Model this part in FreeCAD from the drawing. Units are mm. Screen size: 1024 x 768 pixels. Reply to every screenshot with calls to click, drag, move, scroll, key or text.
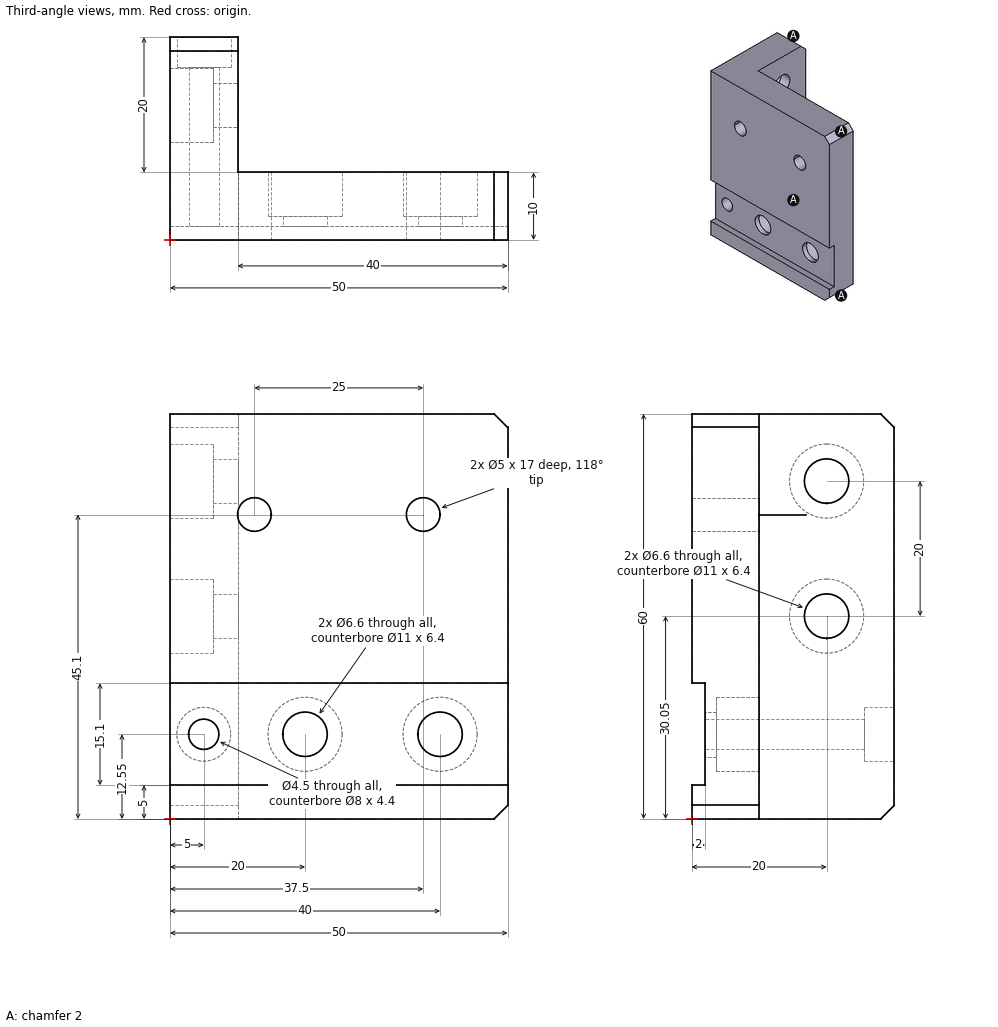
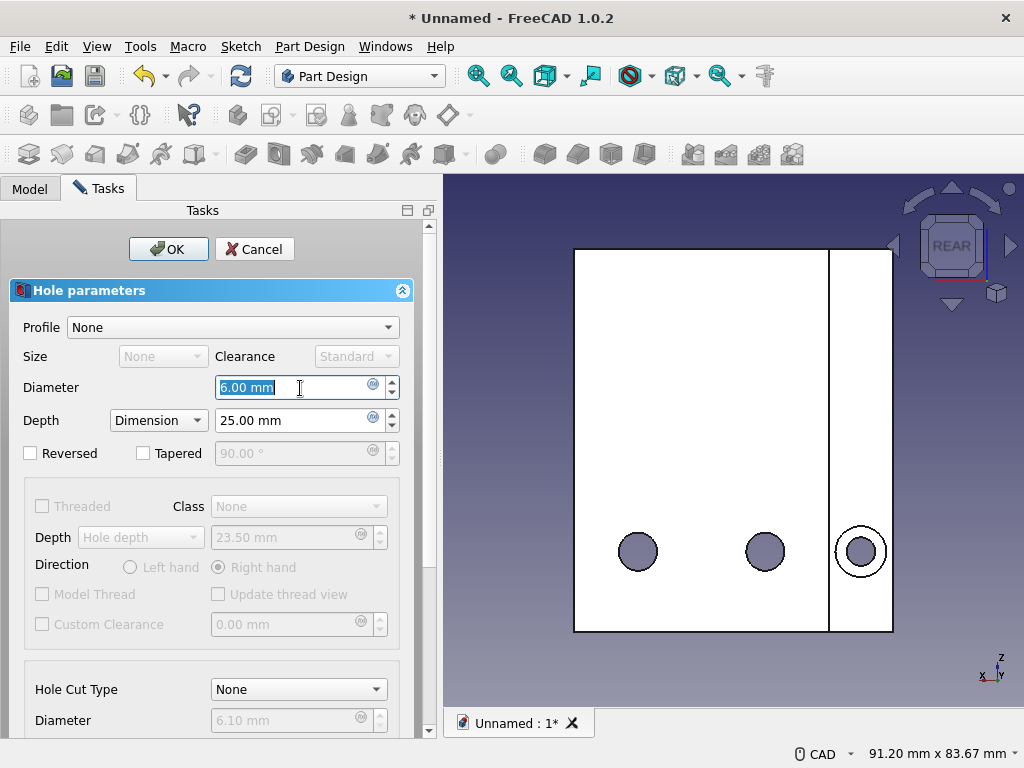
text(6.6)
key(Tab)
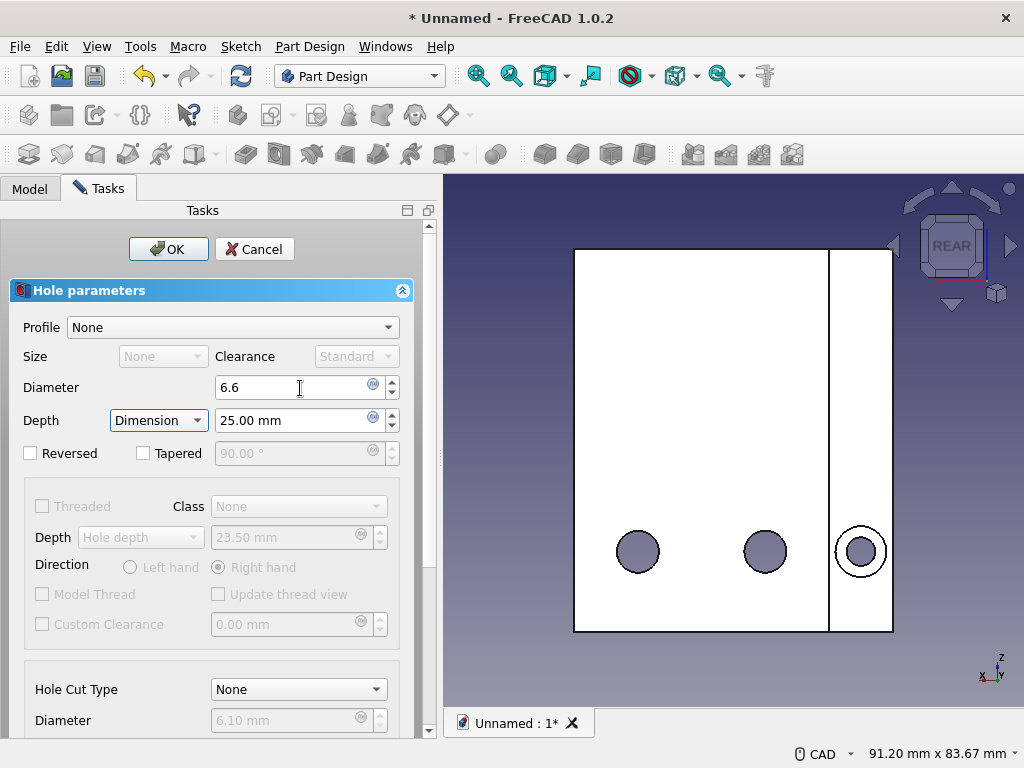
click(160, 420)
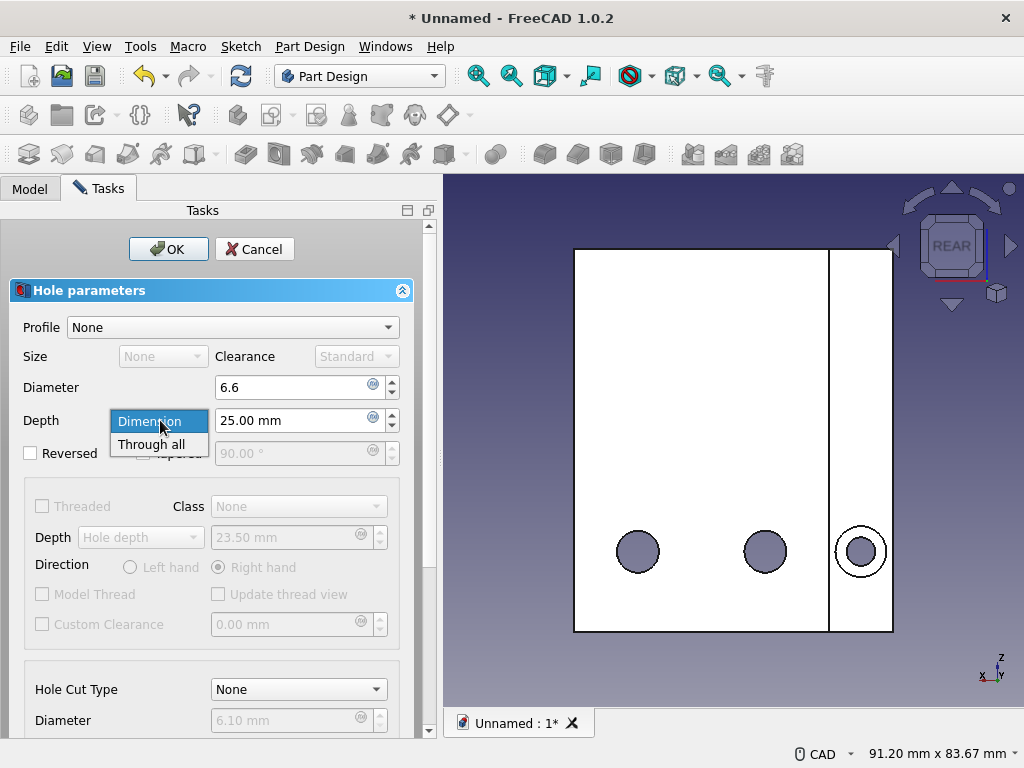
click(158, 444)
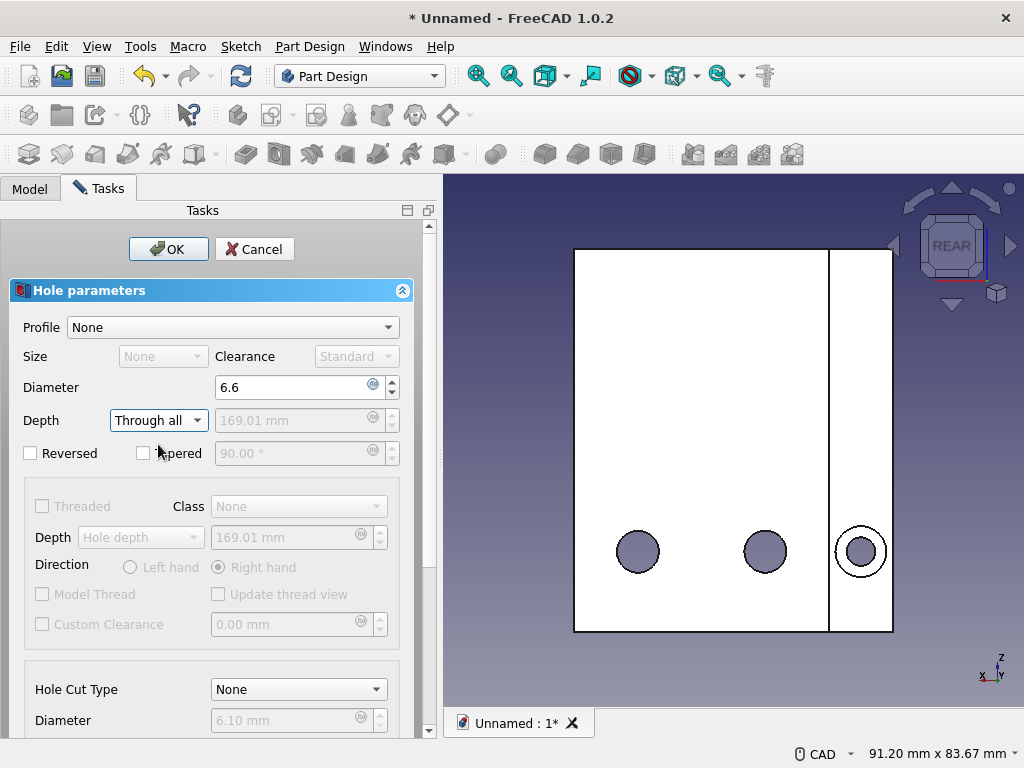
click(300, 690)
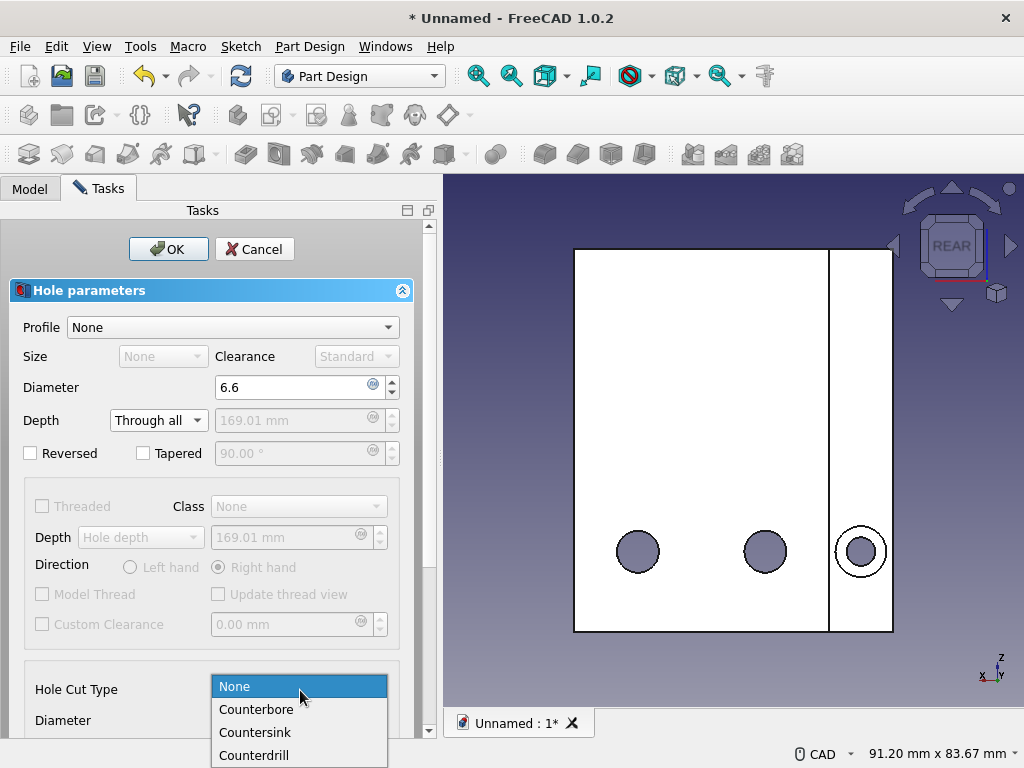
click(298, 710)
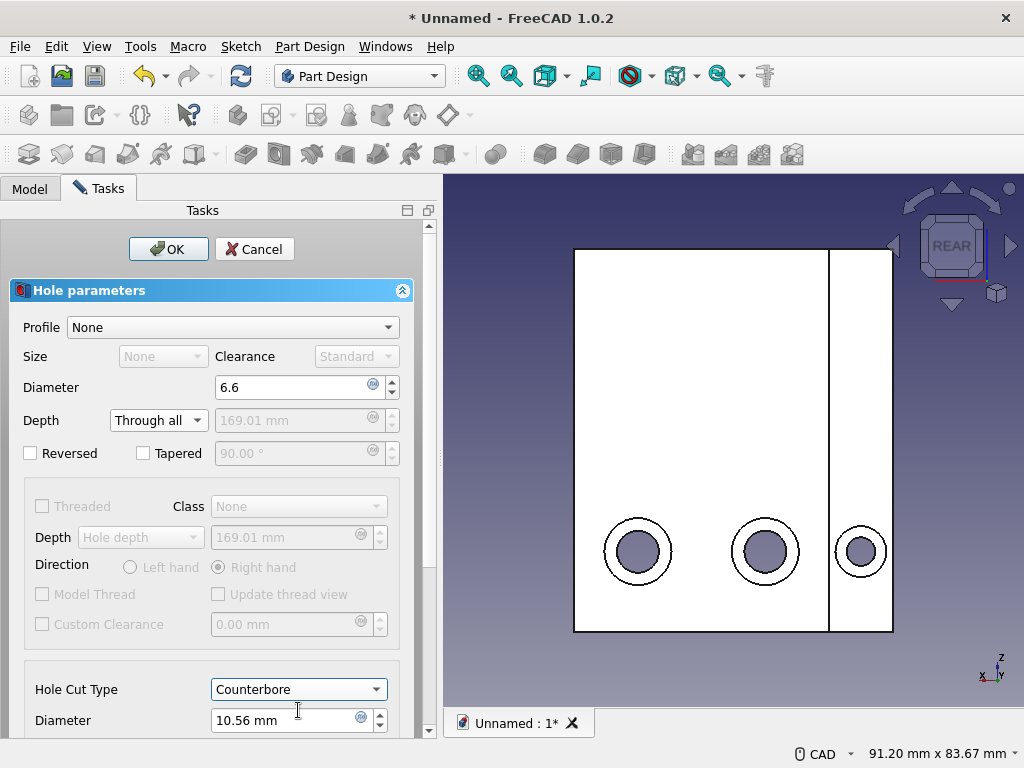
triple_click(292, 720)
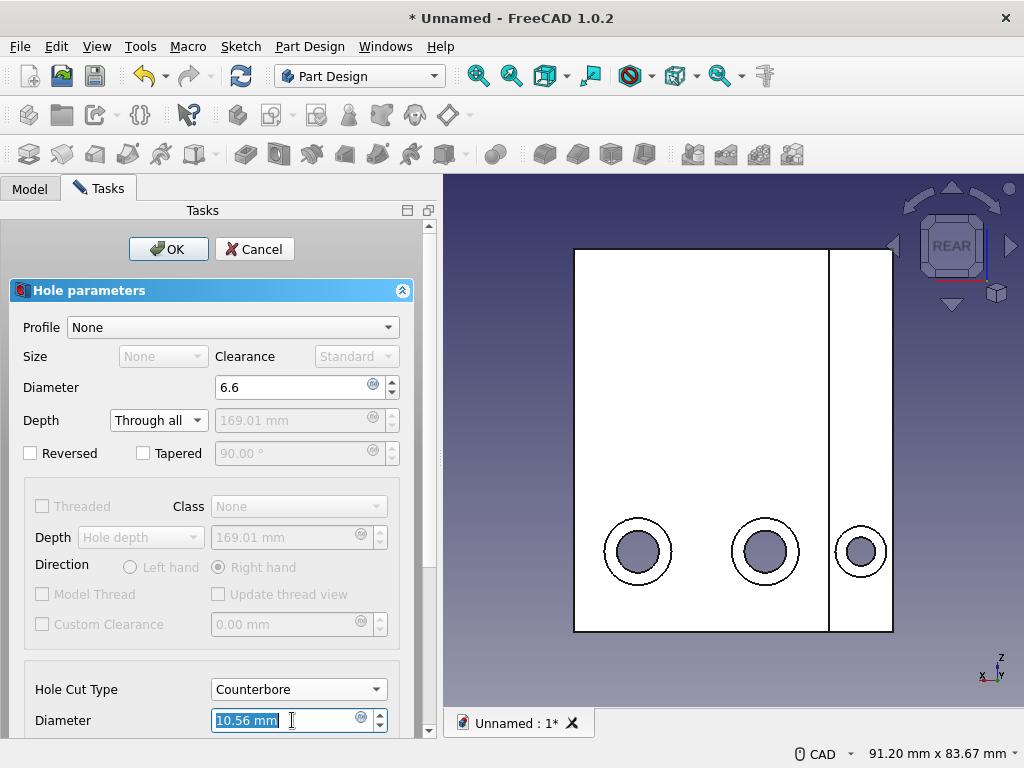
text(11)
key(Tab)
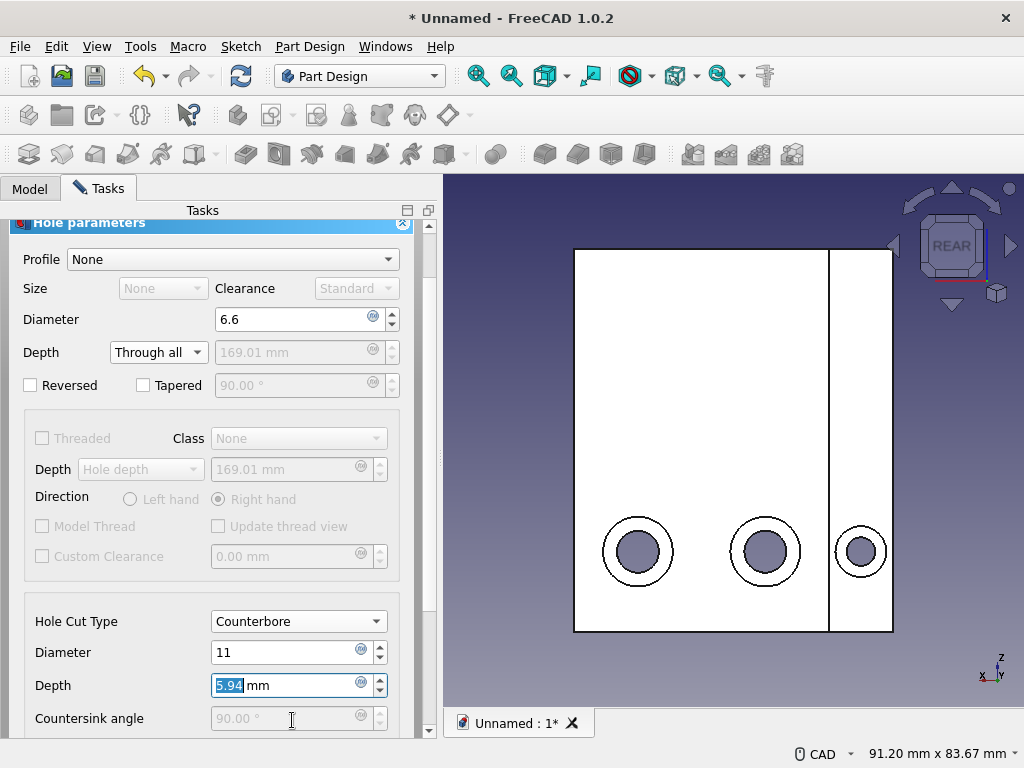
text(6.4)
key(Tab)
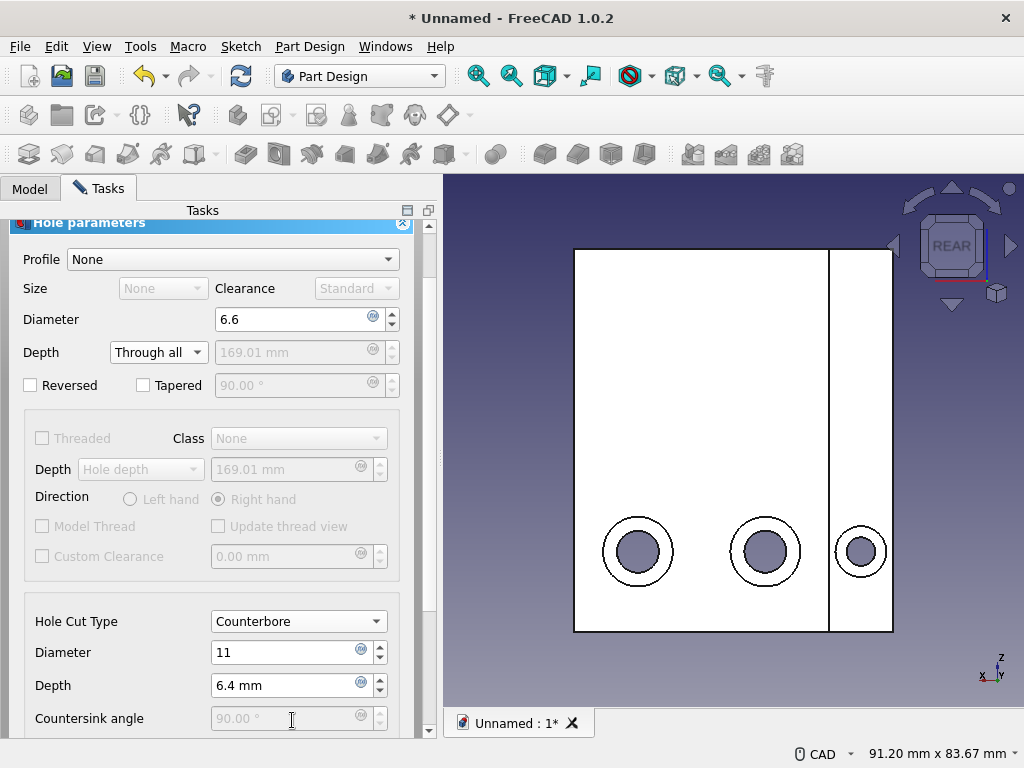
scroll(429, 479, up, 2)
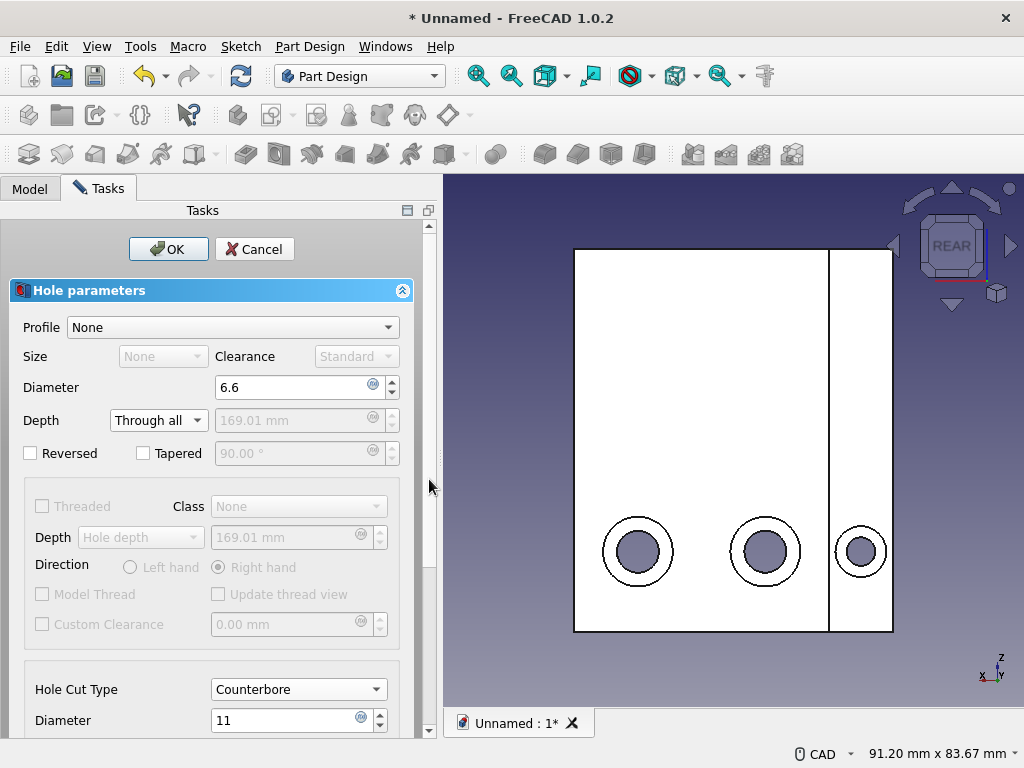
click(169, 249)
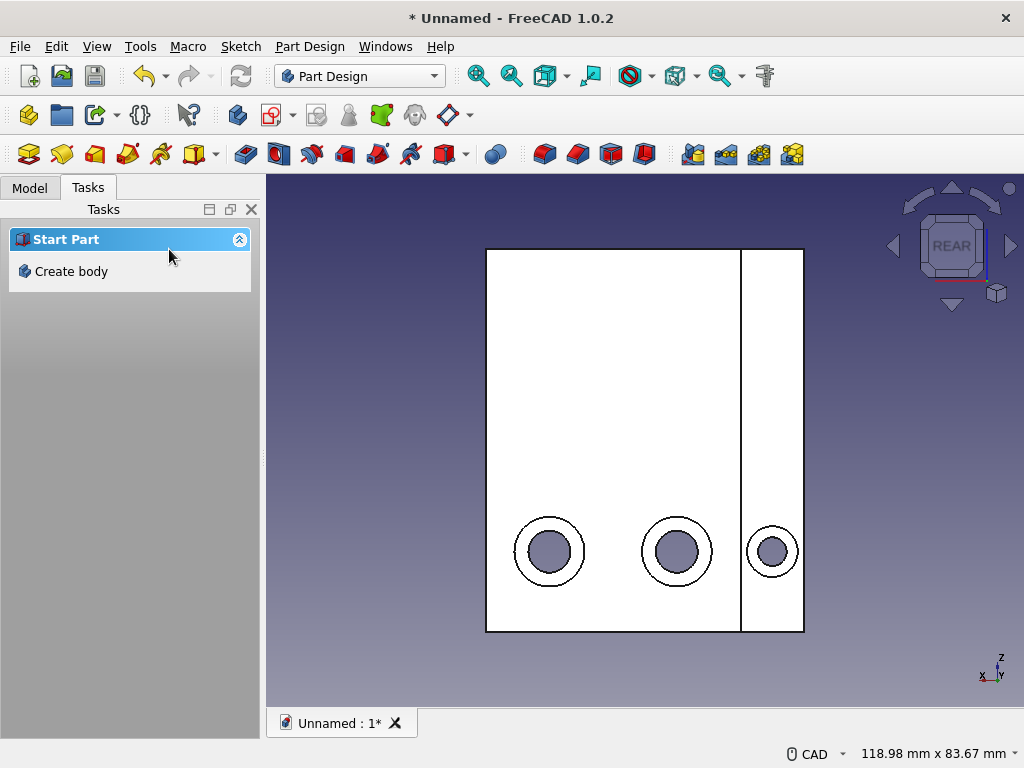
click(270, 116)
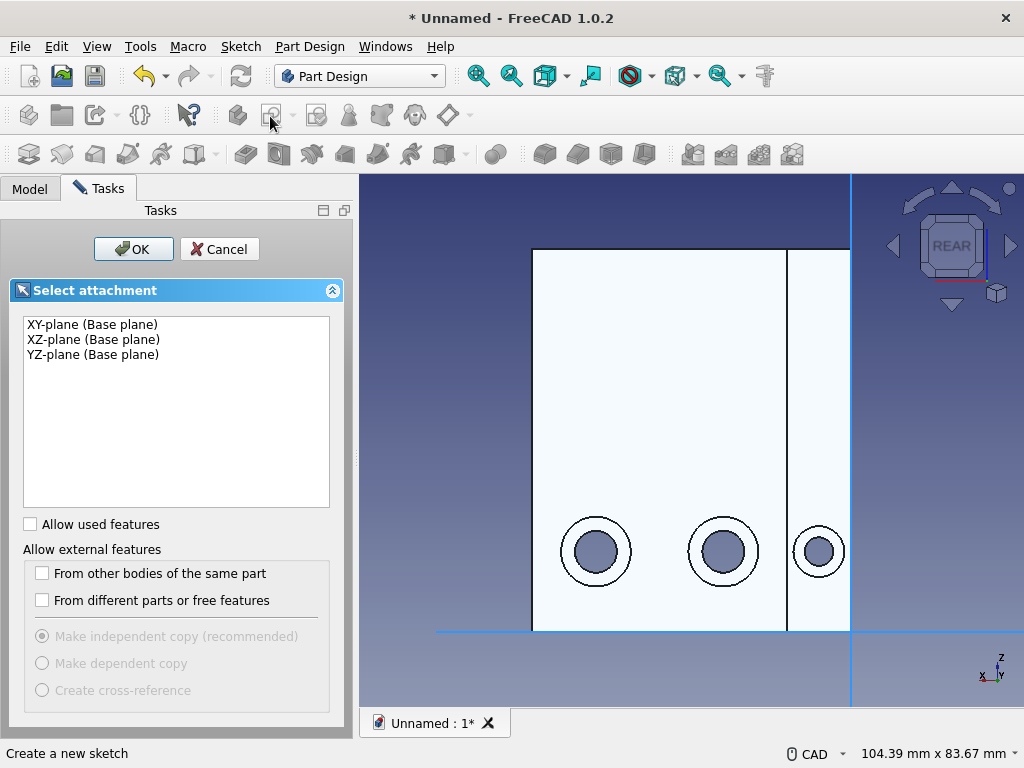
click(84, 354)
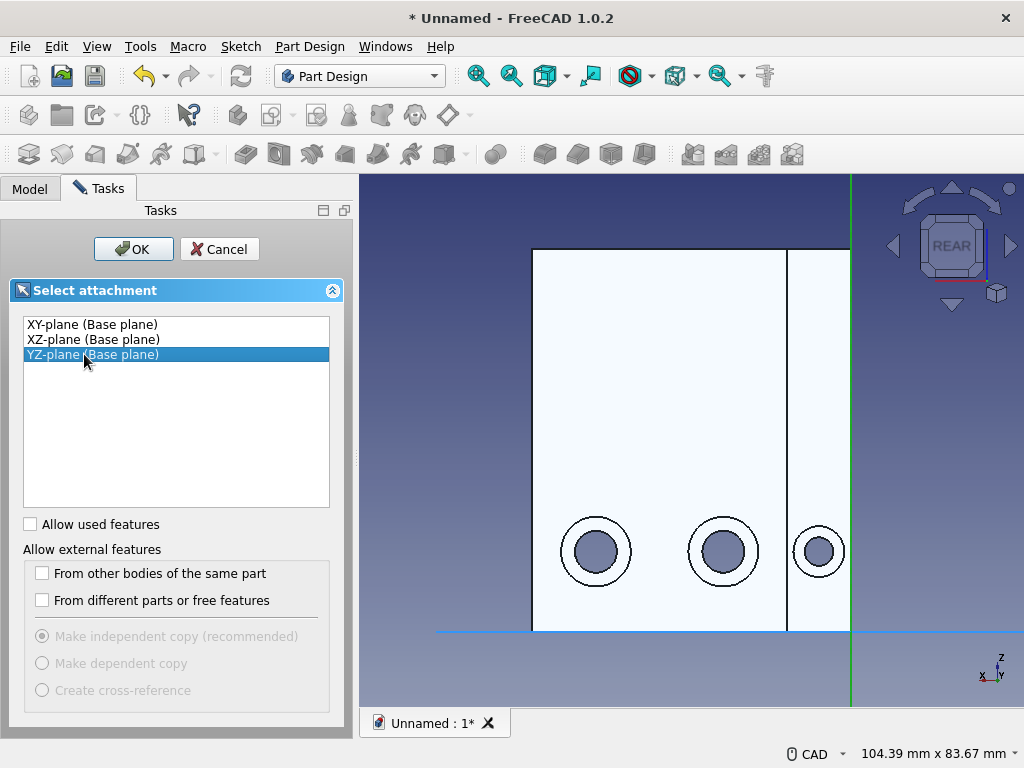
click(134, 249)